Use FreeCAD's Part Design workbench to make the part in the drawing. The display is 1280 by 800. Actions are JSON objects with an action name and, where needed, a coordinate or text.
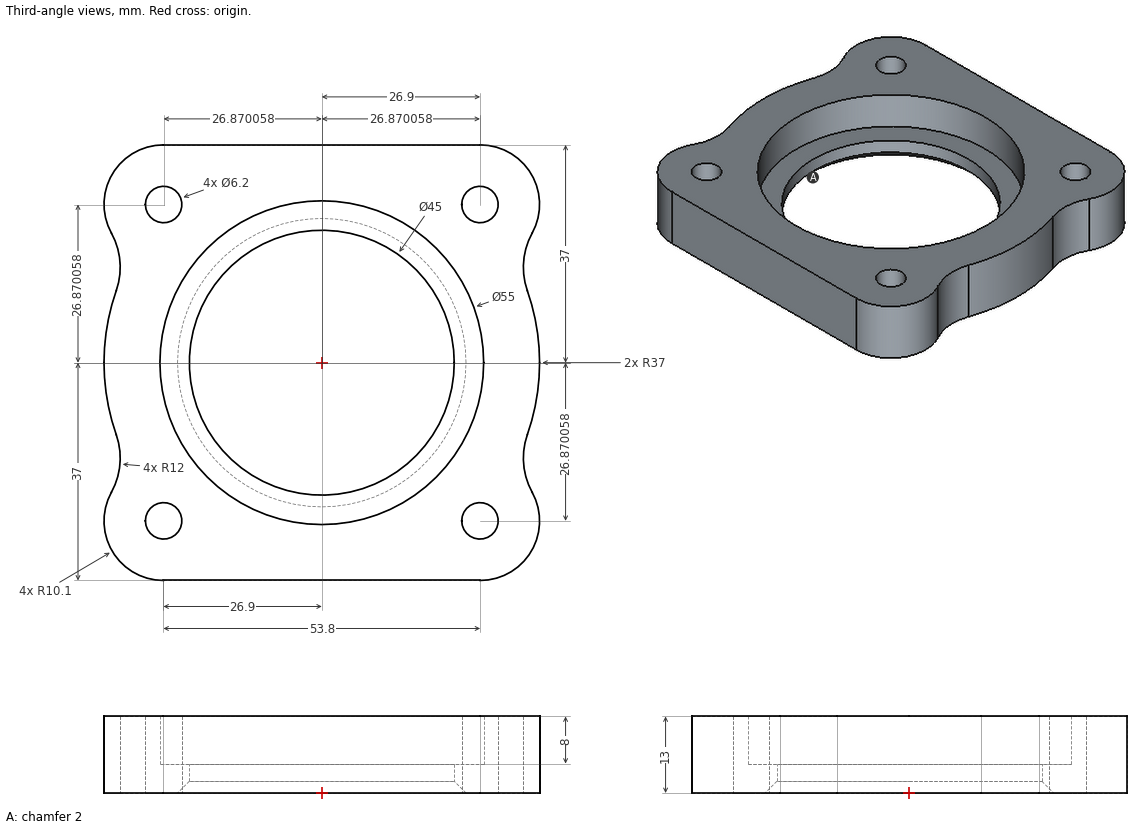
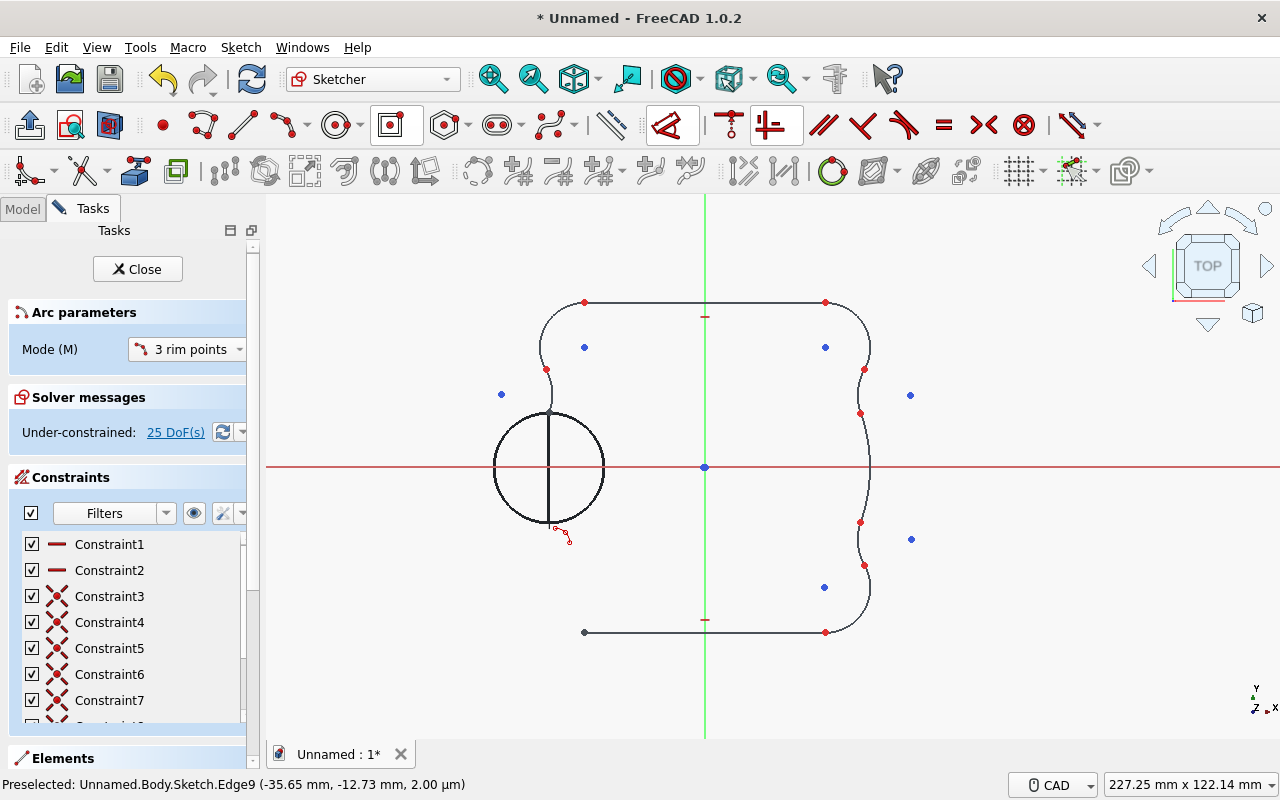
{"action": "scroll", "coordinate": [540, 456], "scroll_direction": "up", "scroll_amount": 3}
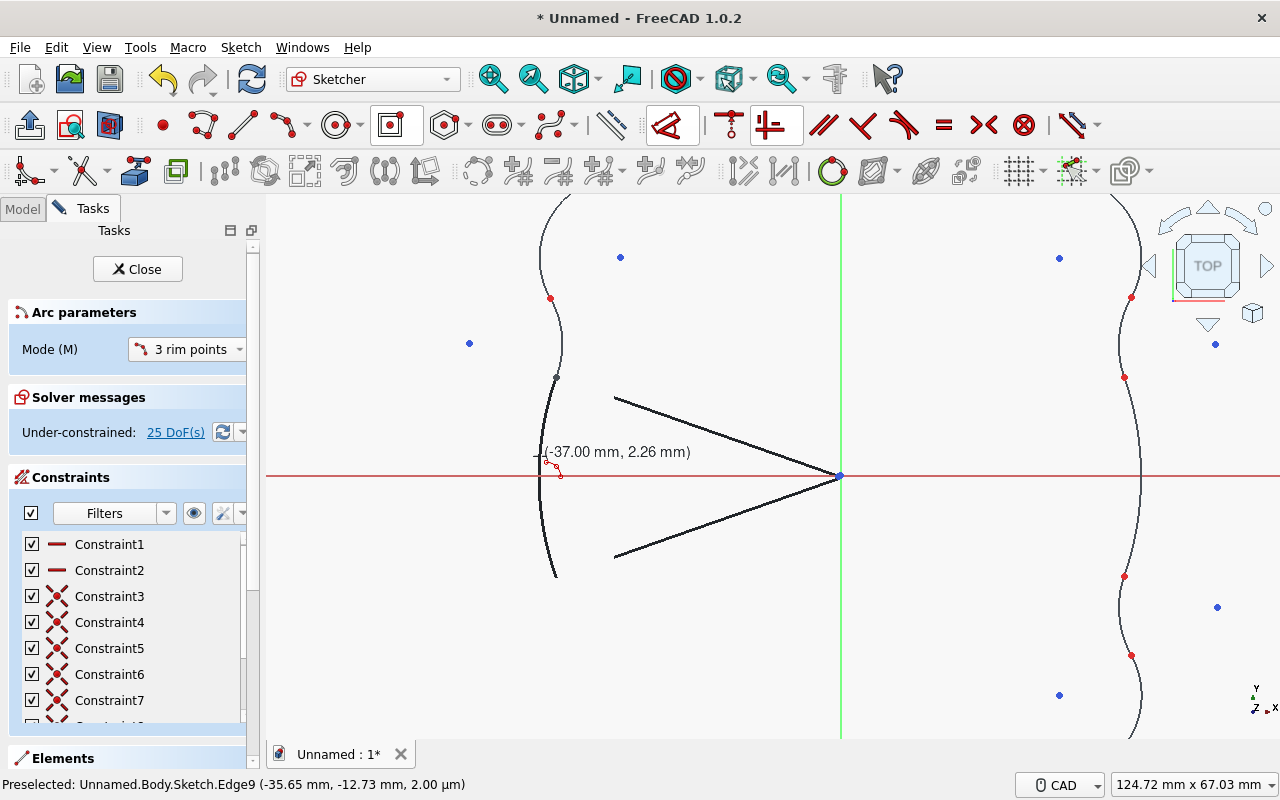
{"action": "left_click", "coordinate": [540, 456]}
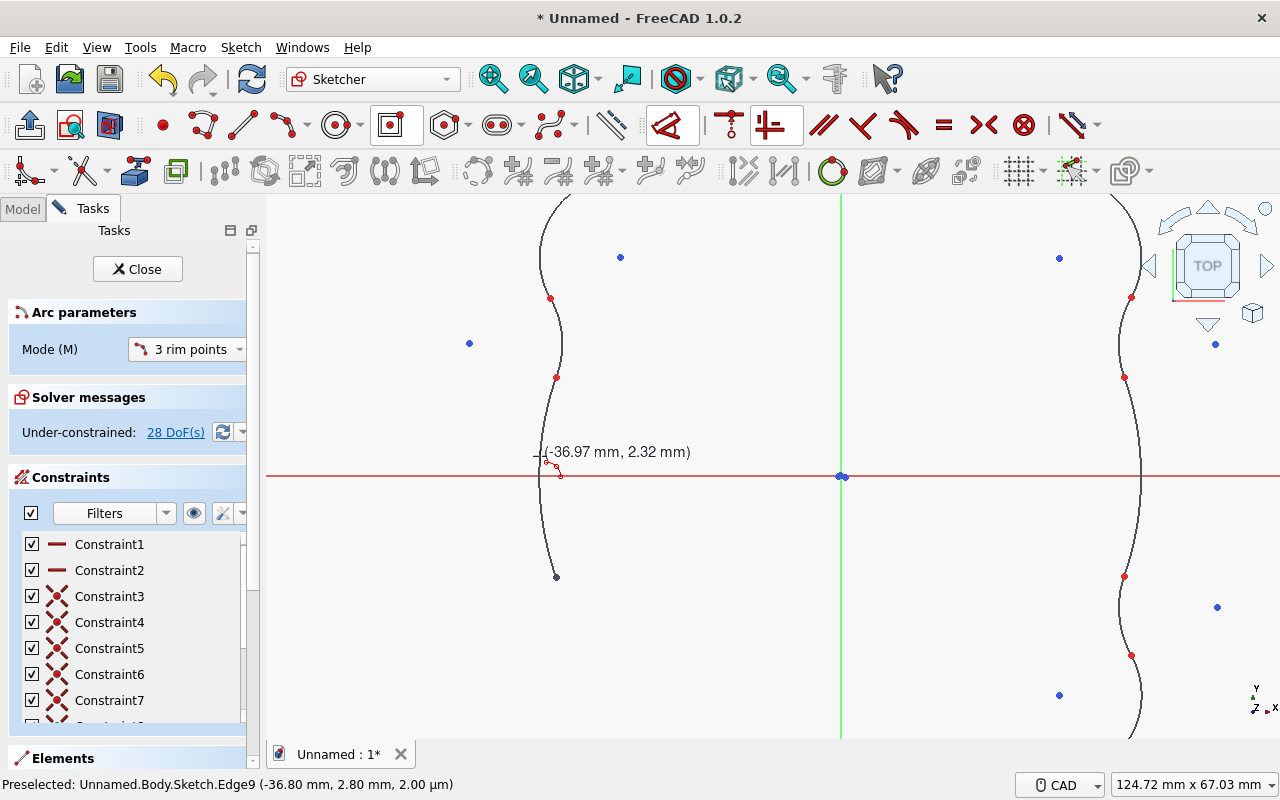
{"action": "left_click", "coordinate": [556, 578]}
{"action": "left_click", "coordinate": [550, 655]}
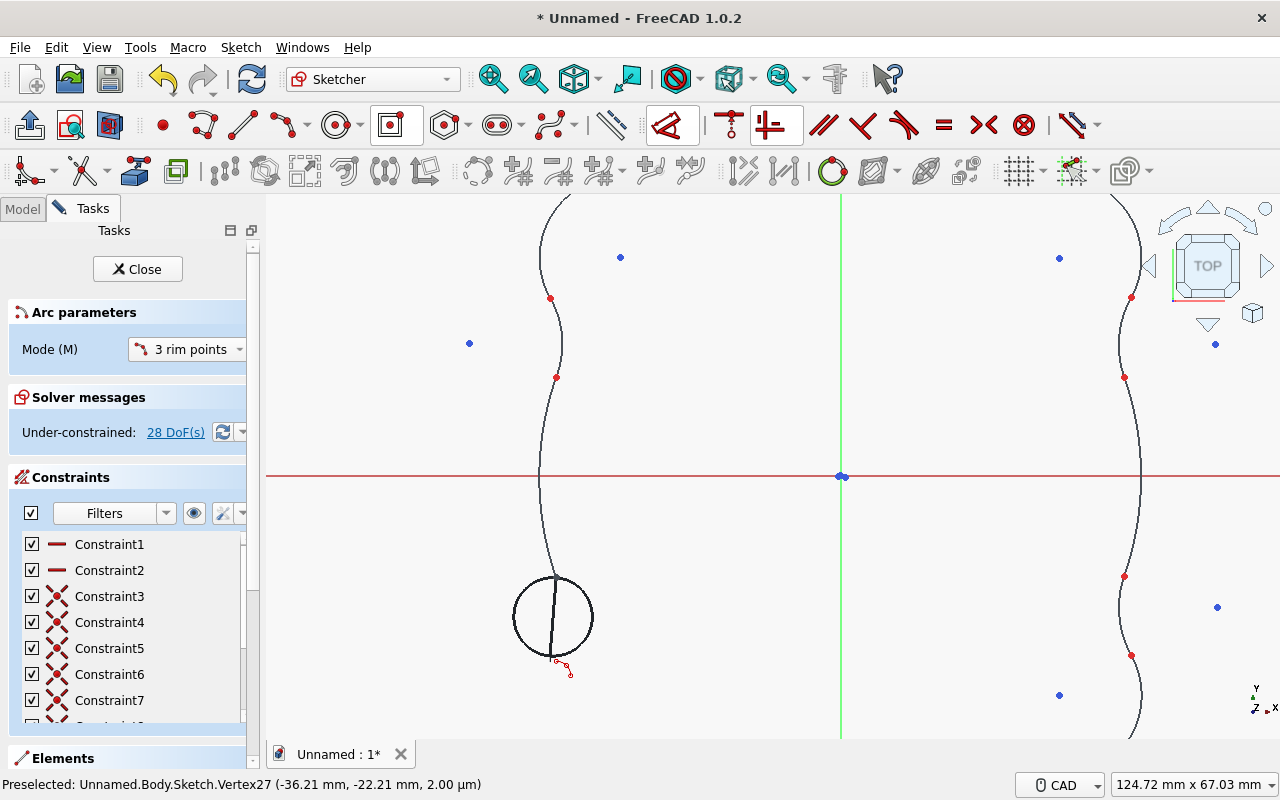
{"action": "scroll", "coordinate": [562, 616], "scroll_direction": "up", "scroll_amount": 4}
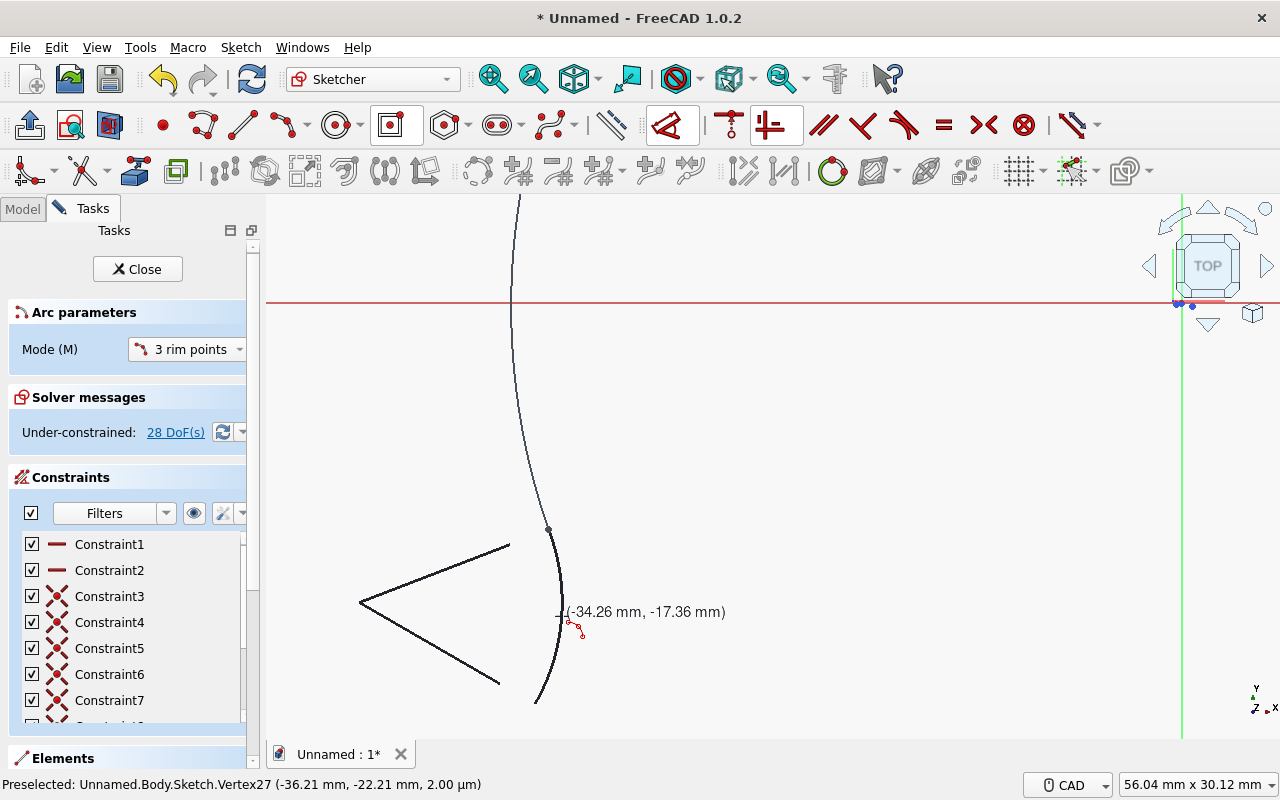
{"action": "left_click", "coordinate": [561, 615]}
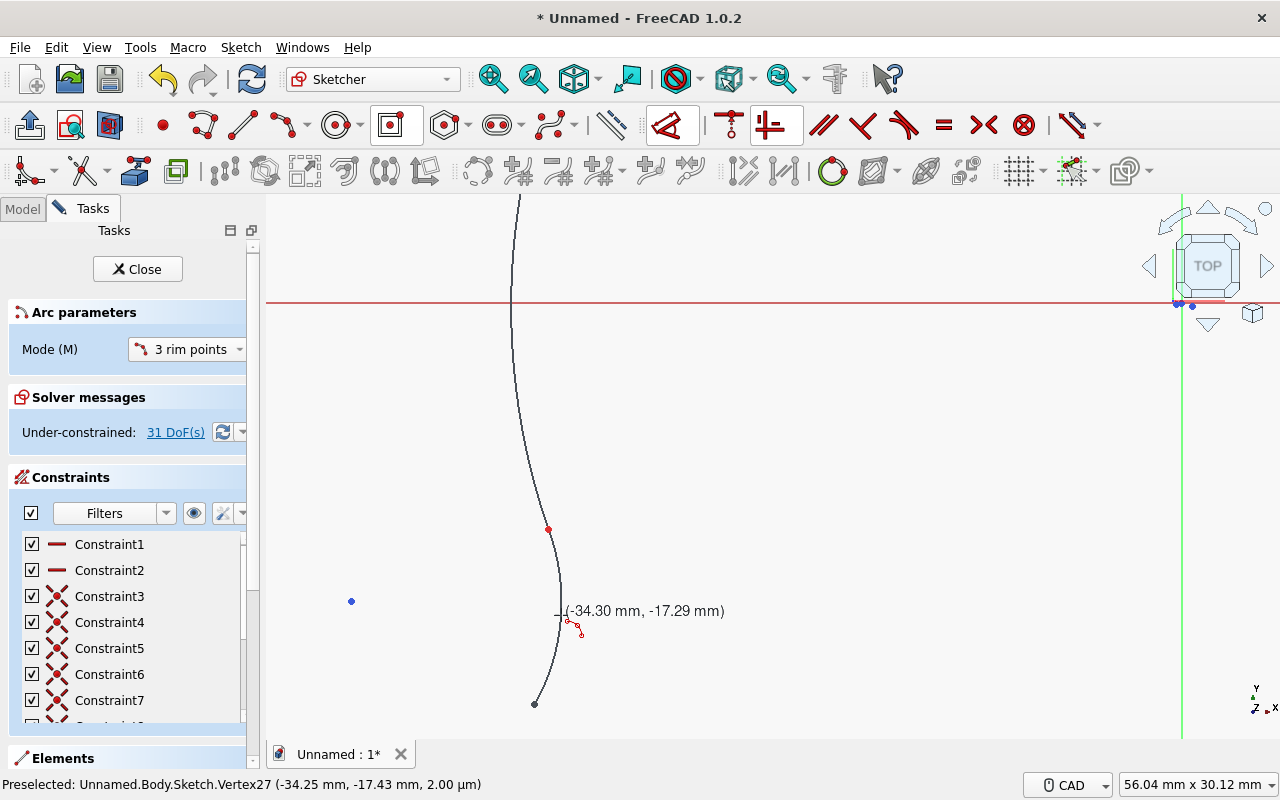
{"action": "left_click", "coordinate": [535, 704]}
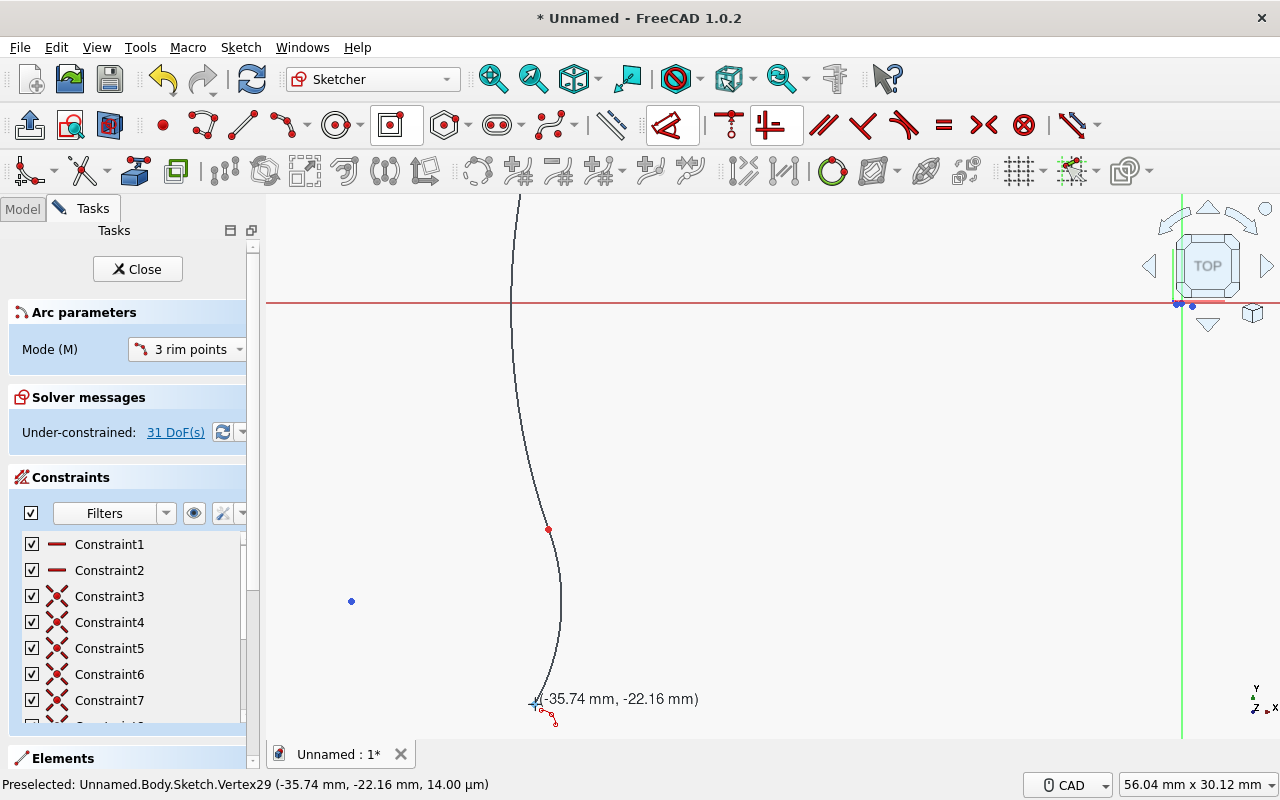
{"action": "scroll", "coordinate": [548, 520], "scroll_direction": "down", "scroll_amount": 7}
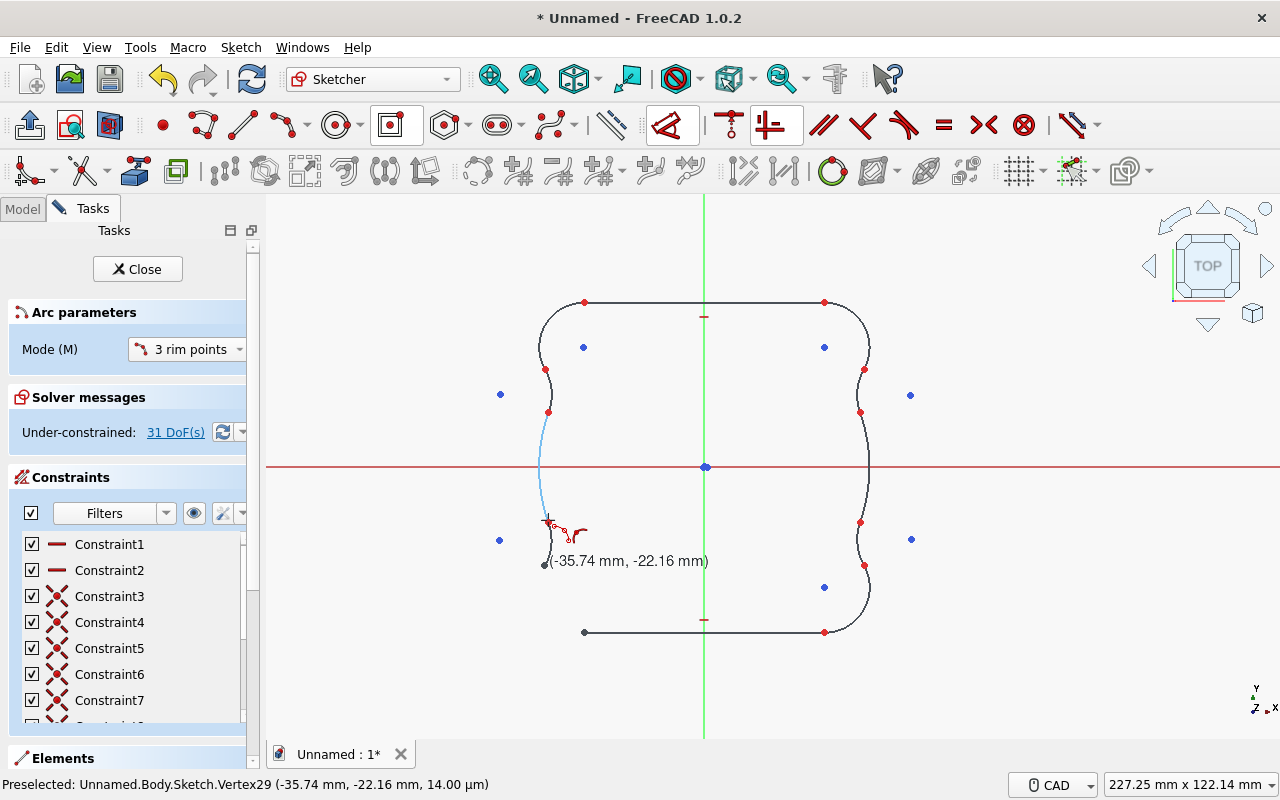
{"action": "left_click", "coordinate": [584, 633]}
{"action": "left_click", "coordinate": [546, 610]}
{"action": "key", "text": "Escape"}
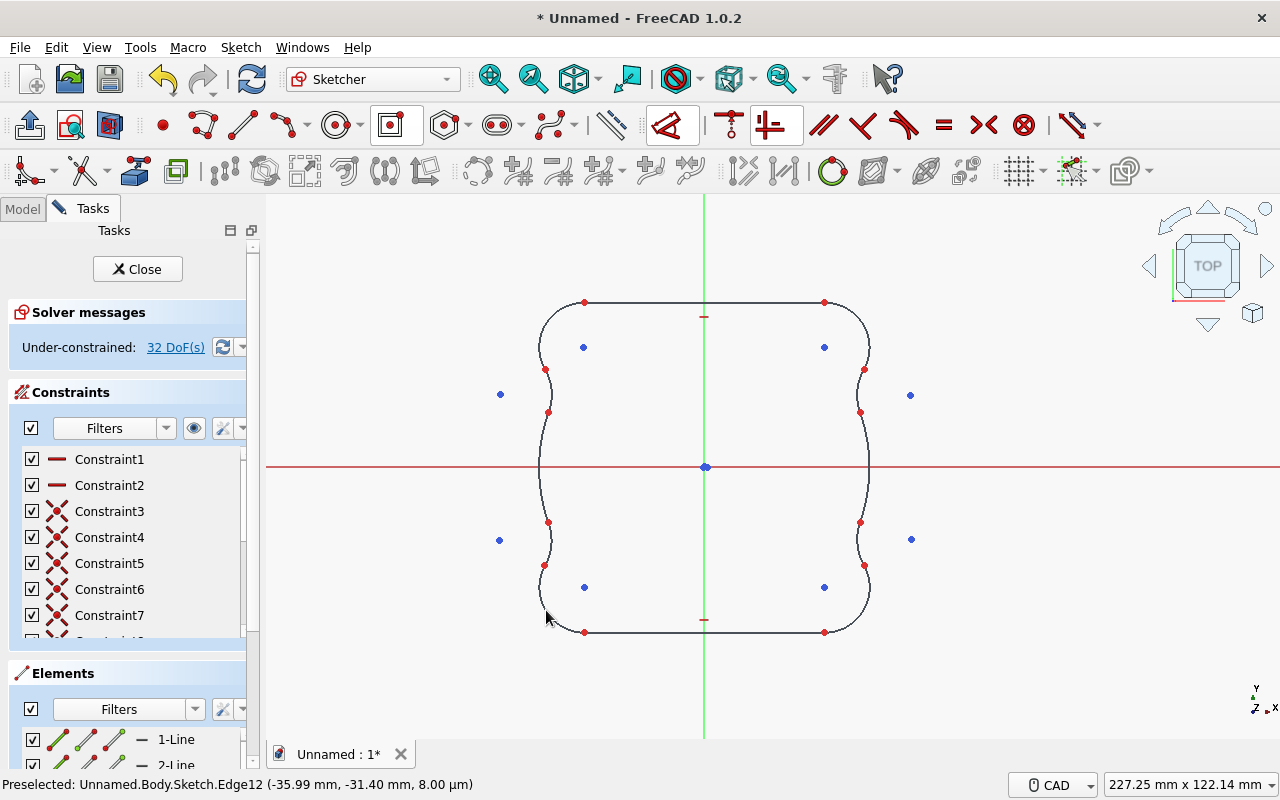
{"action": "left_click", "coordinate": [656, 633]}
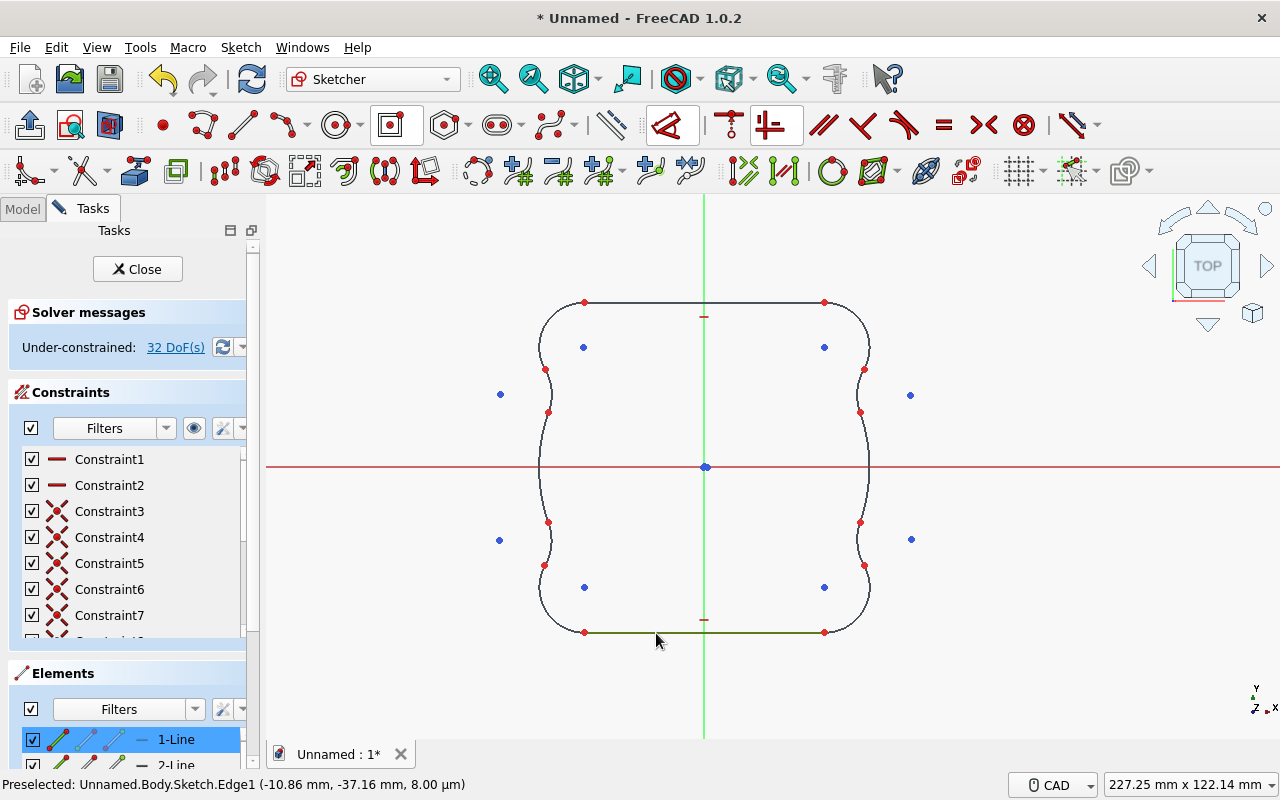
{"action": "left_click", "coordinate": [851, 624]}